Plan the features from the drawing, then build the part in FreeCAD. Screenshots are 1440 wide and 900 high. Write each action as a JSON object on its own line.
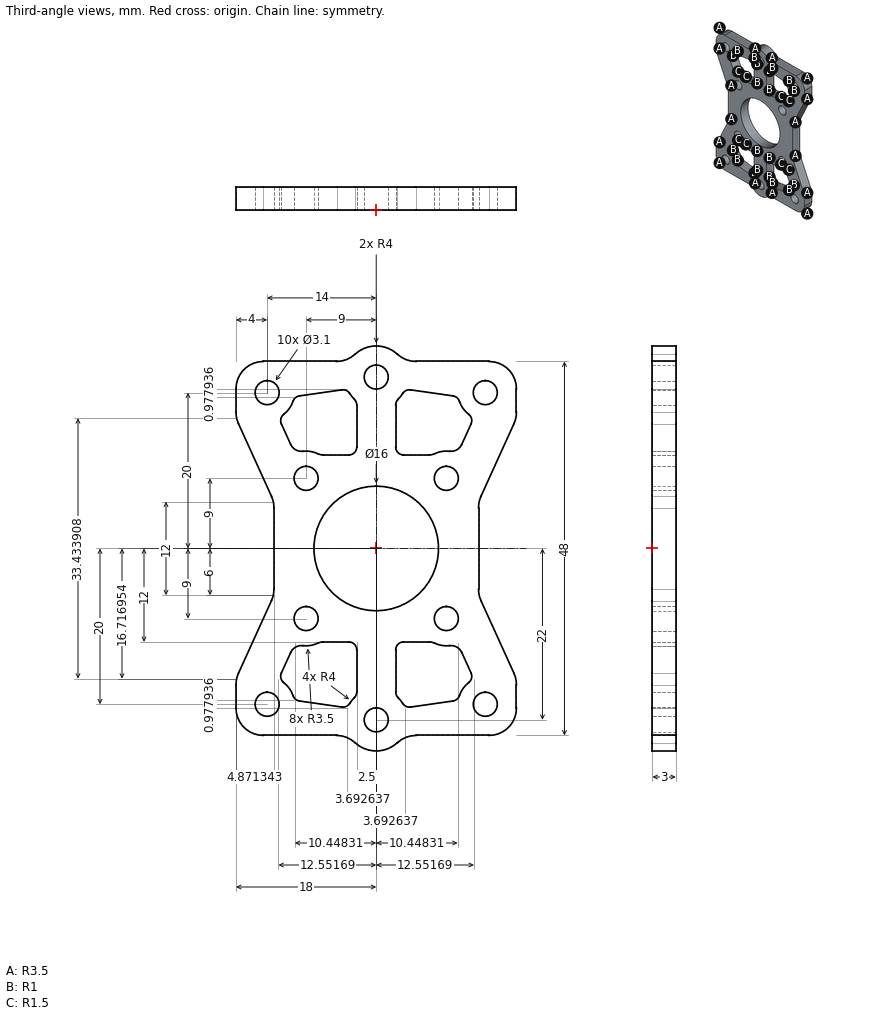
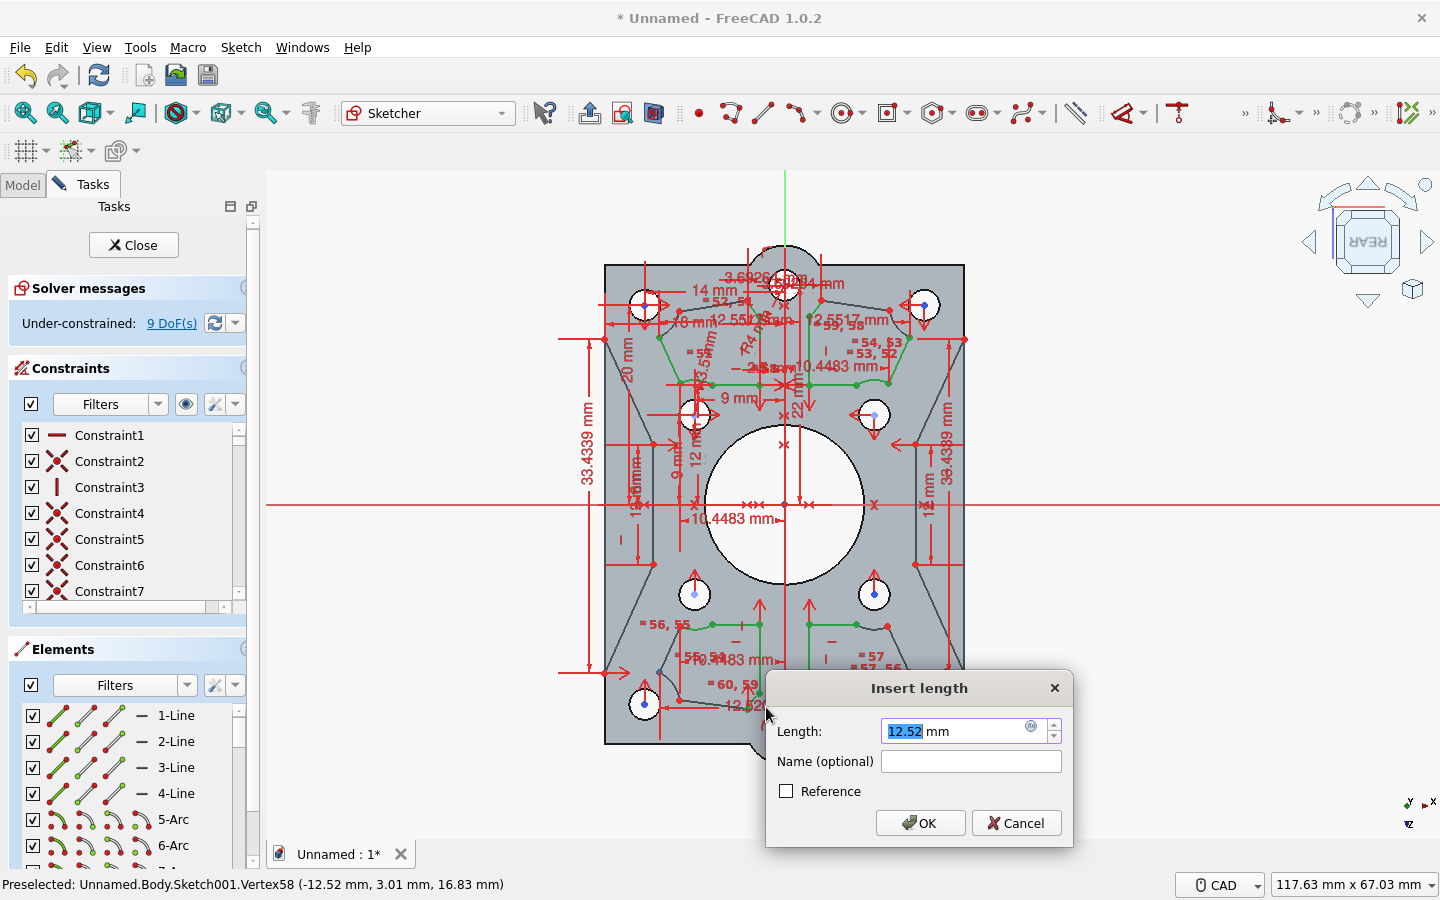
{"action": "type", "text": "12.55169"}
{"action": "key", "text": "Return"}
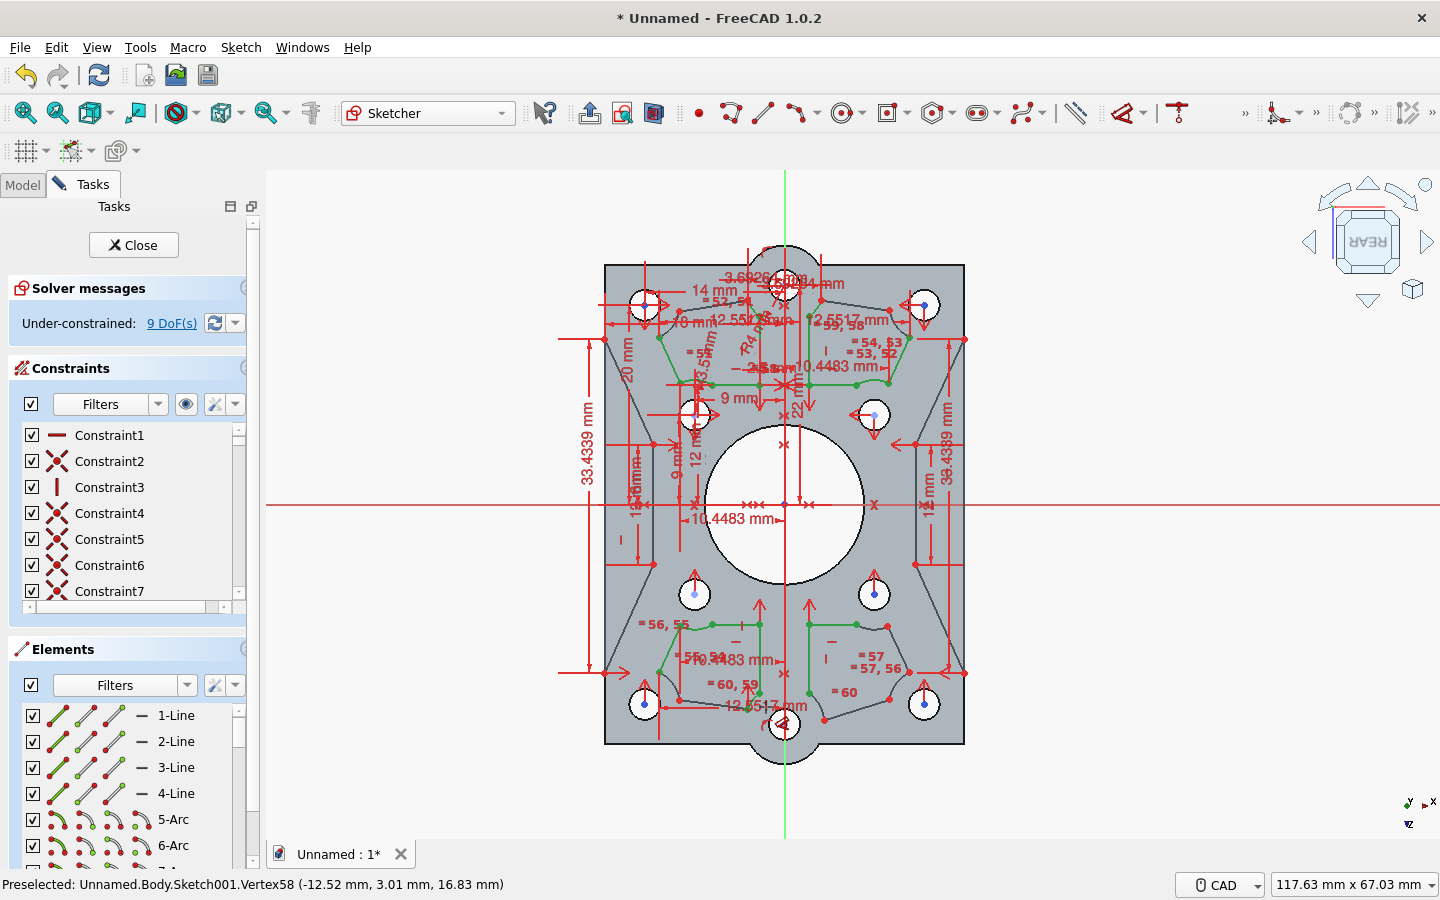
{"action": "left_click", "coordinate": [824, 720]}
{"action": "left_click", "coordinate": [804, 754]}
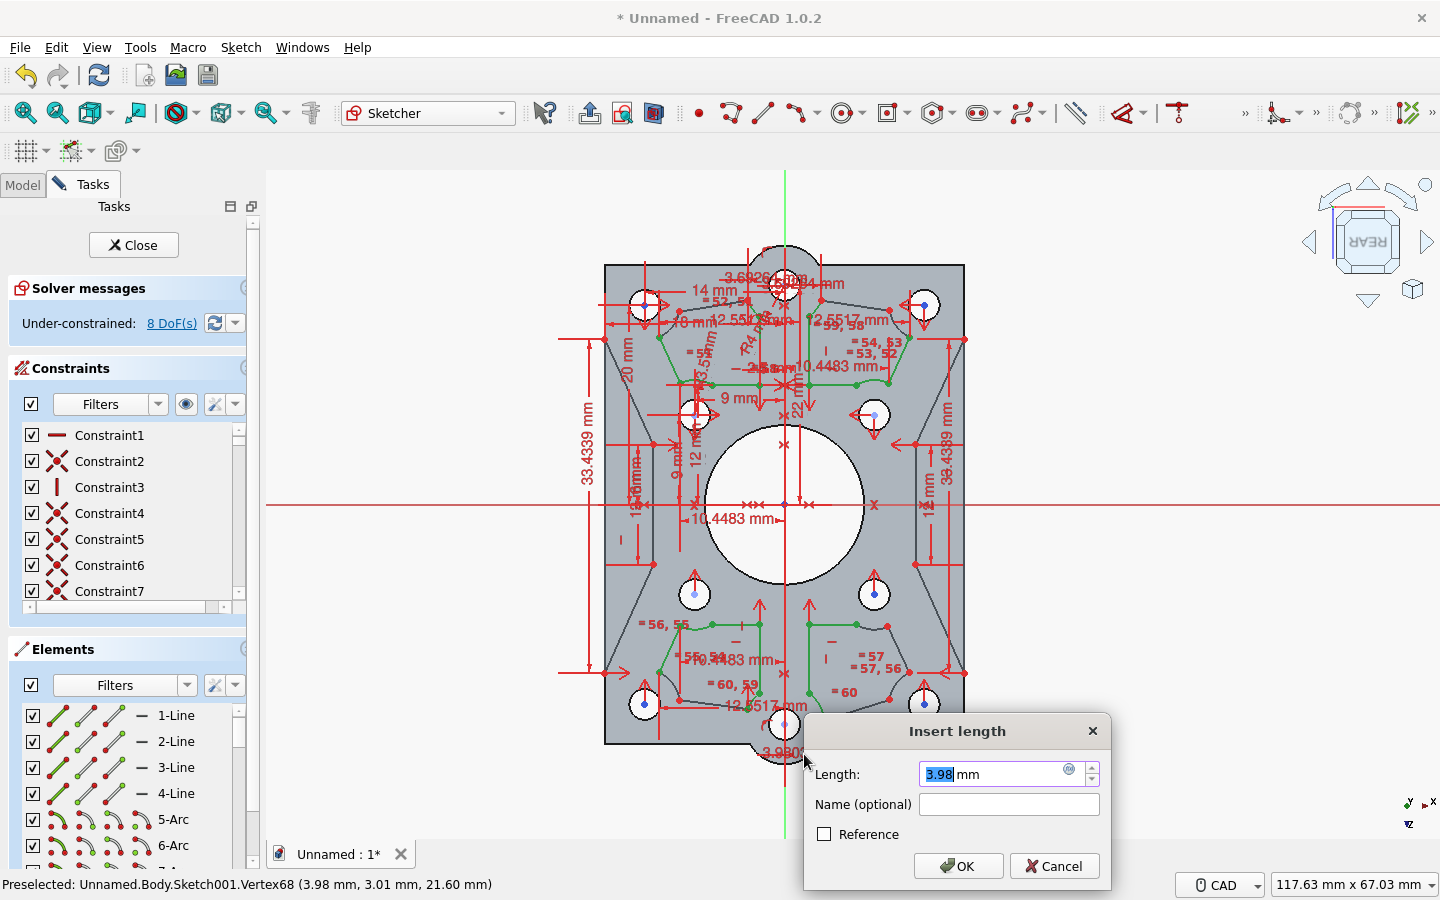
{"action": "type", "text": "3.692637"}
{"action": "key", "text": "Return"}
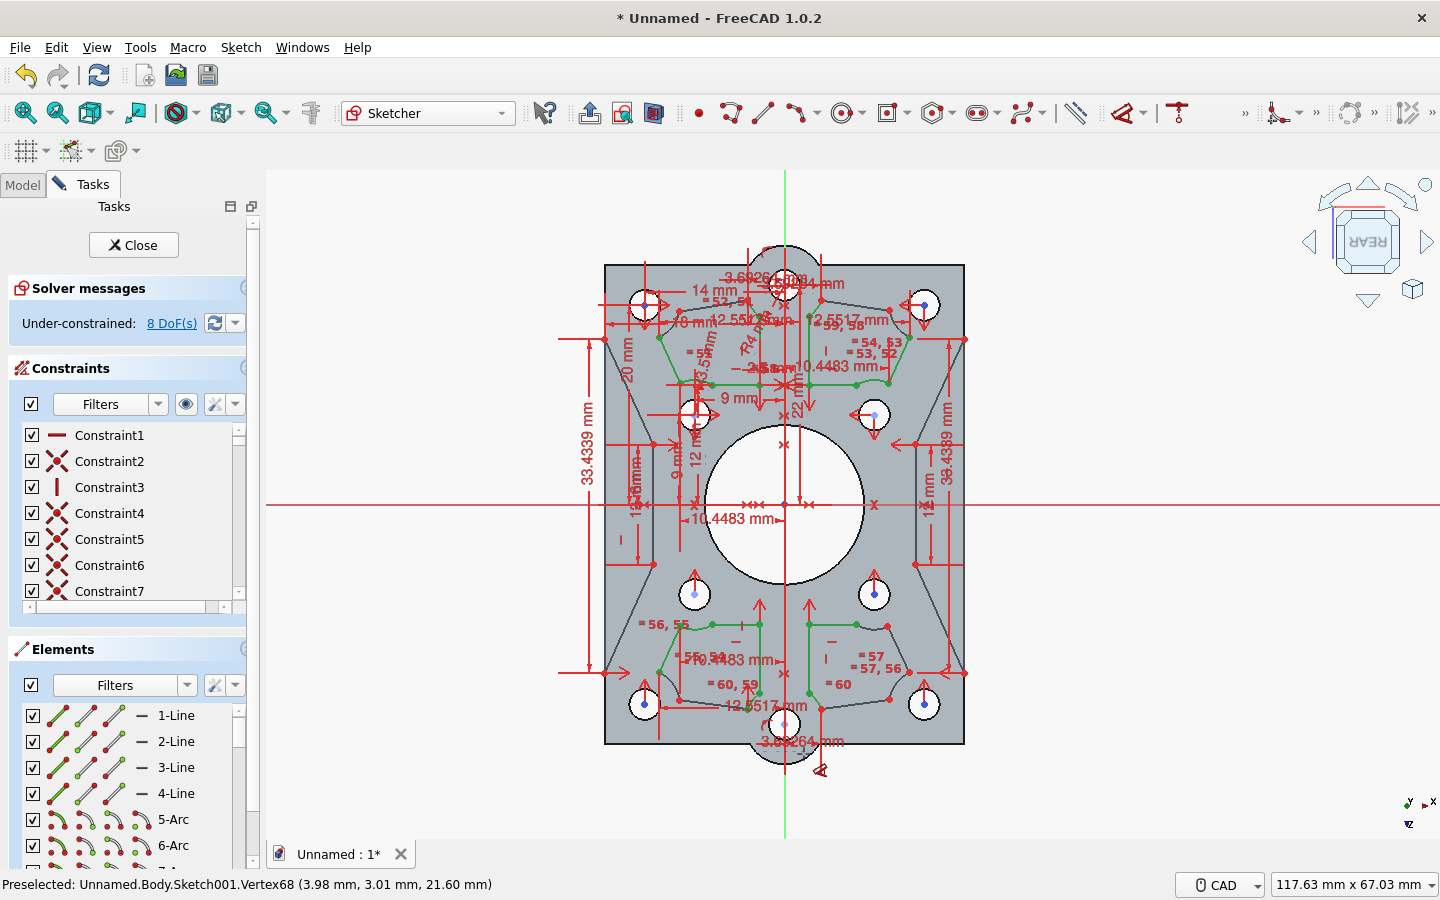
{"action": "left_click", "coordinate": [909, 673]}
{"action": "left_click", "coordinate": [847, 471]}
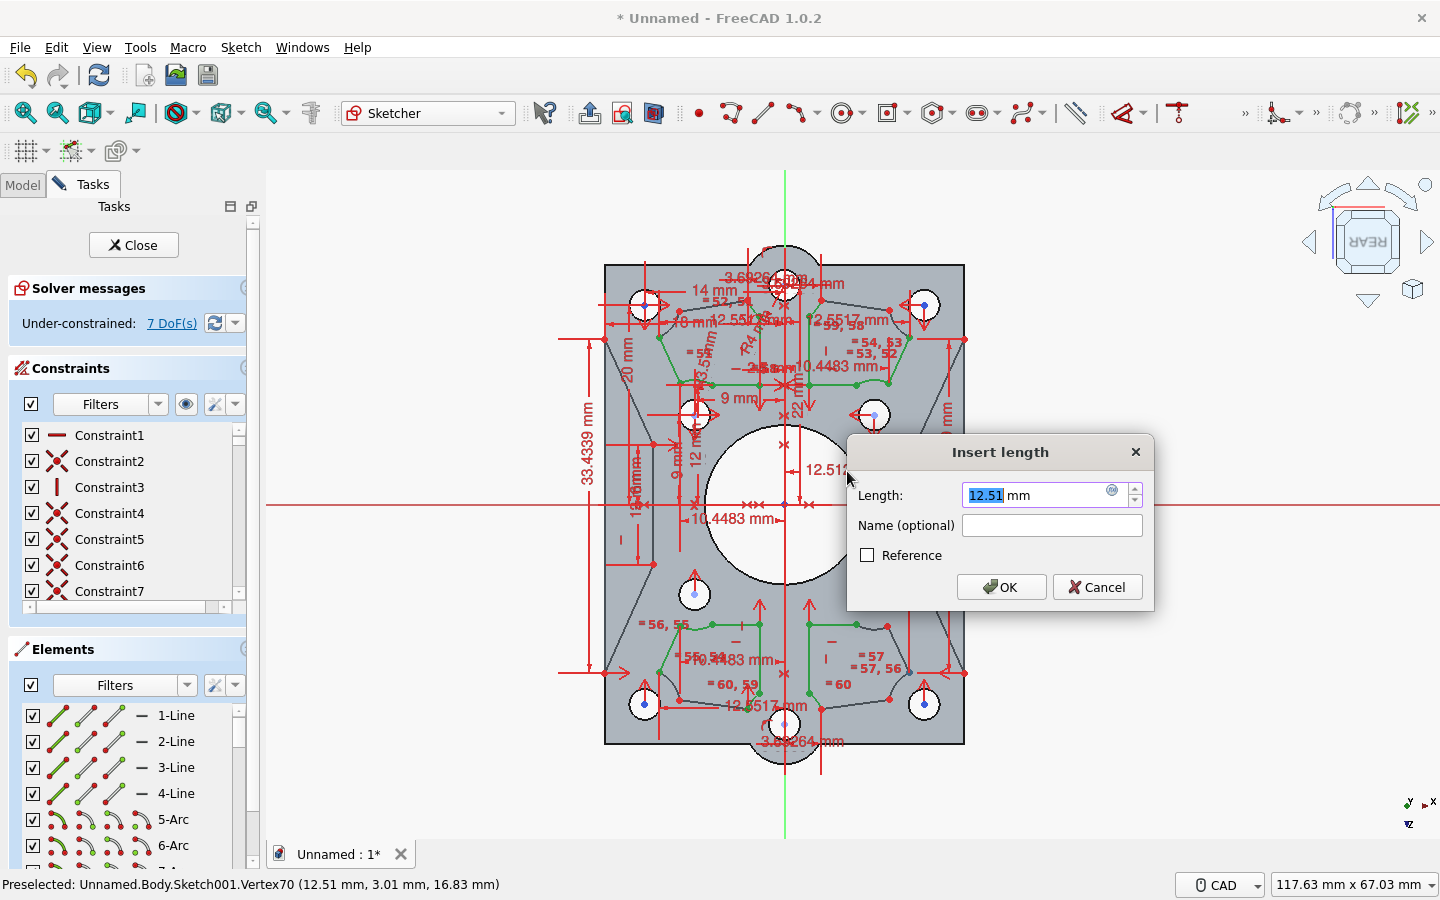
{"action": "type", "text": "12.55169"}
{"action": "key", "text": "Return"}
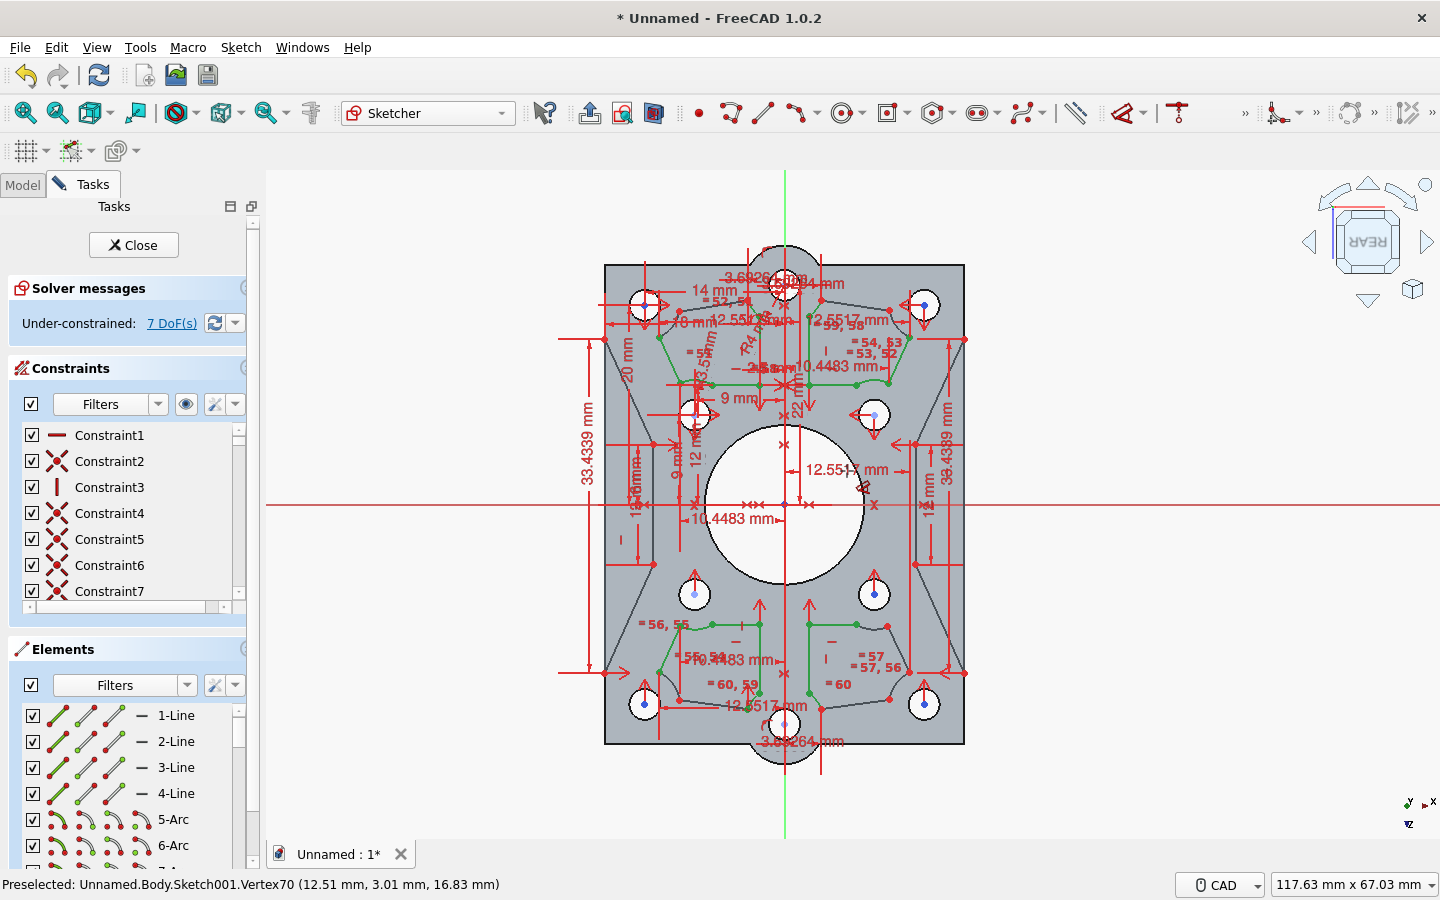
{"action": "left_click", "coordinate": [888, 627]}
{"action": "left_click", "coordinate": [836, 661]}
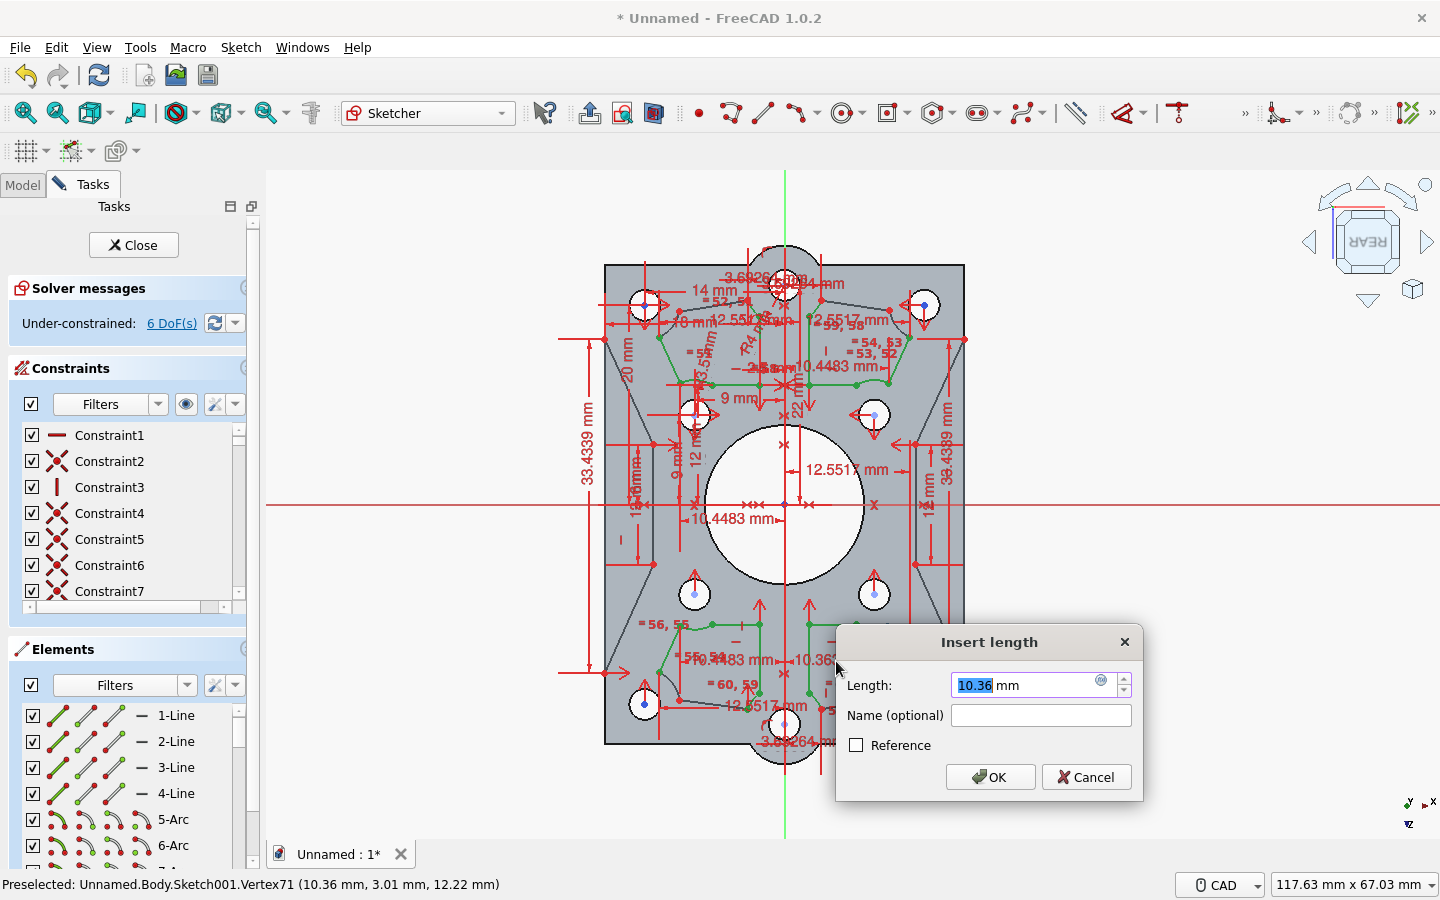
{"action": "type", "text": "10.44831"}
{"action": "key", "text": "Return"}